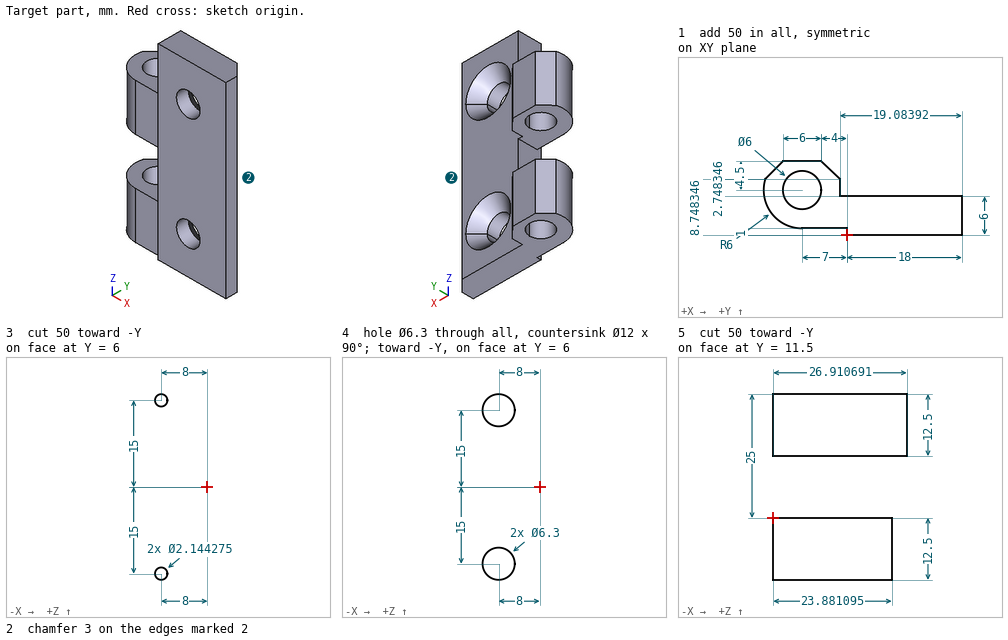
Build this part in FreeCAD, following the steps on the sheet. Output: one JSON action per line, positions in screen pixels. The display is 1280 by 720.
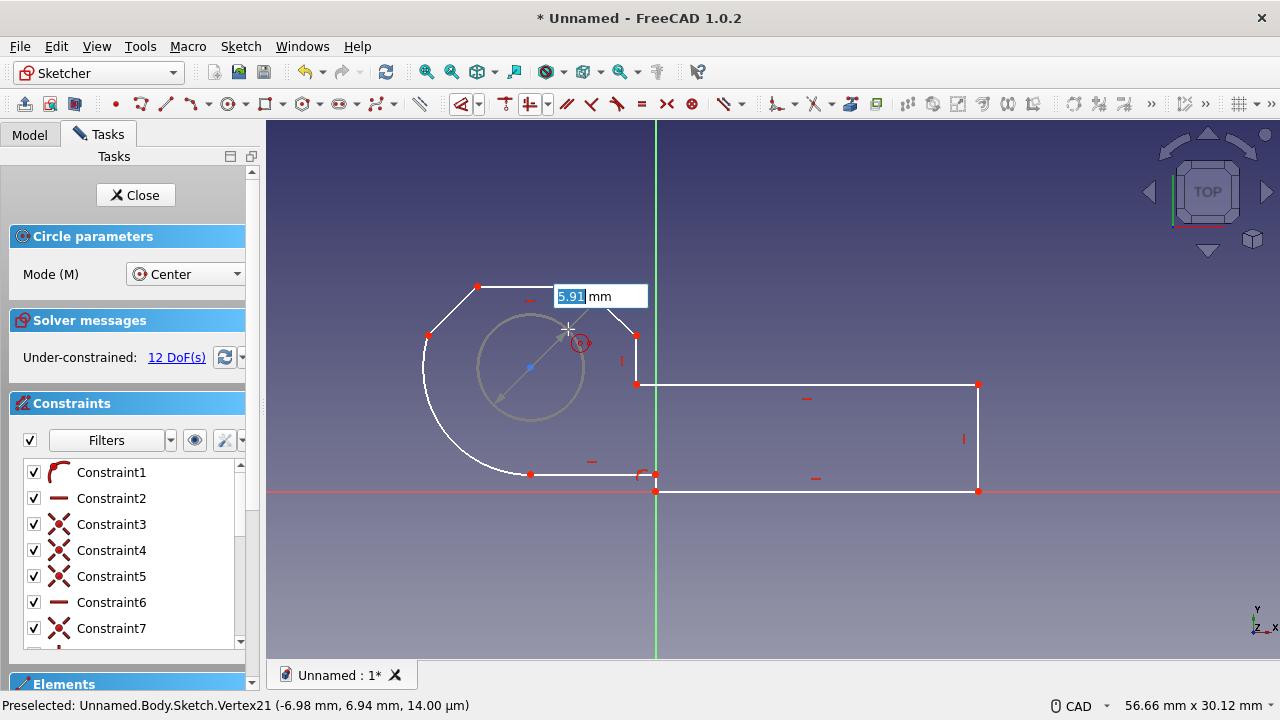
{"action": "type", "text": "6"}
{"action": "key", "text": "Return"}
{"action": "key", "text": "Escape"}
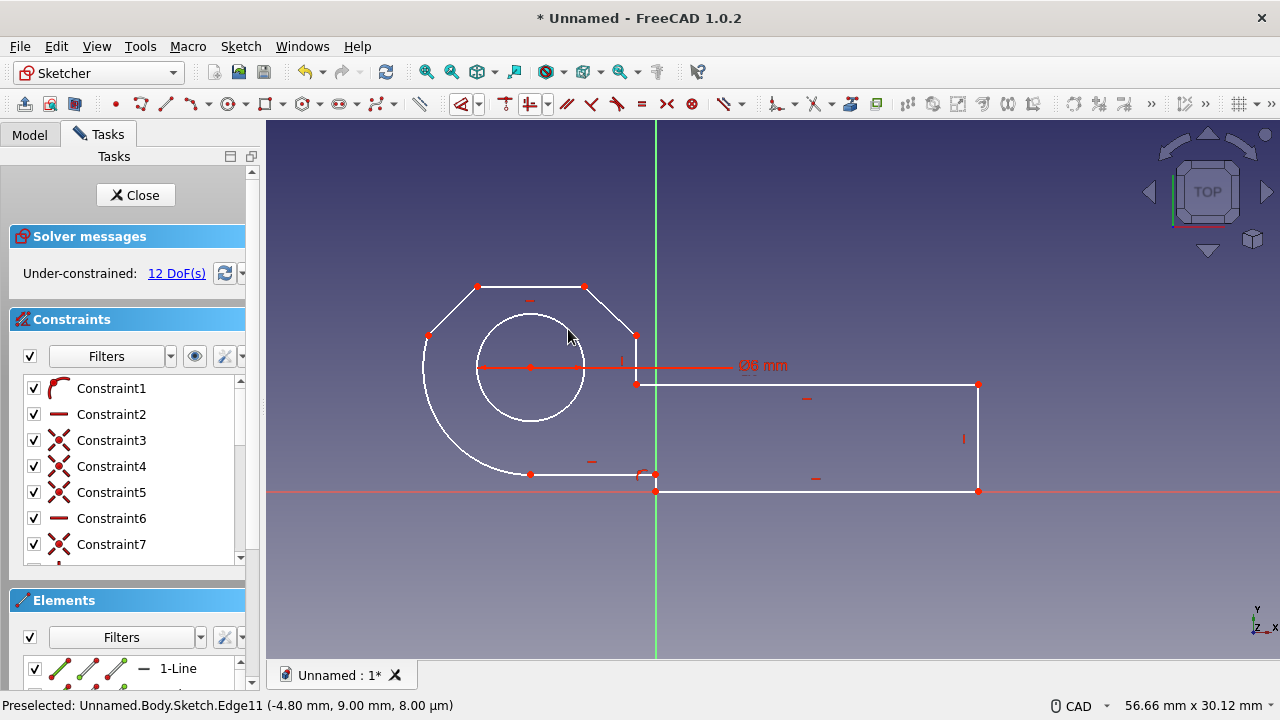
{"action": "left_click", "coordinate": [568, 475]}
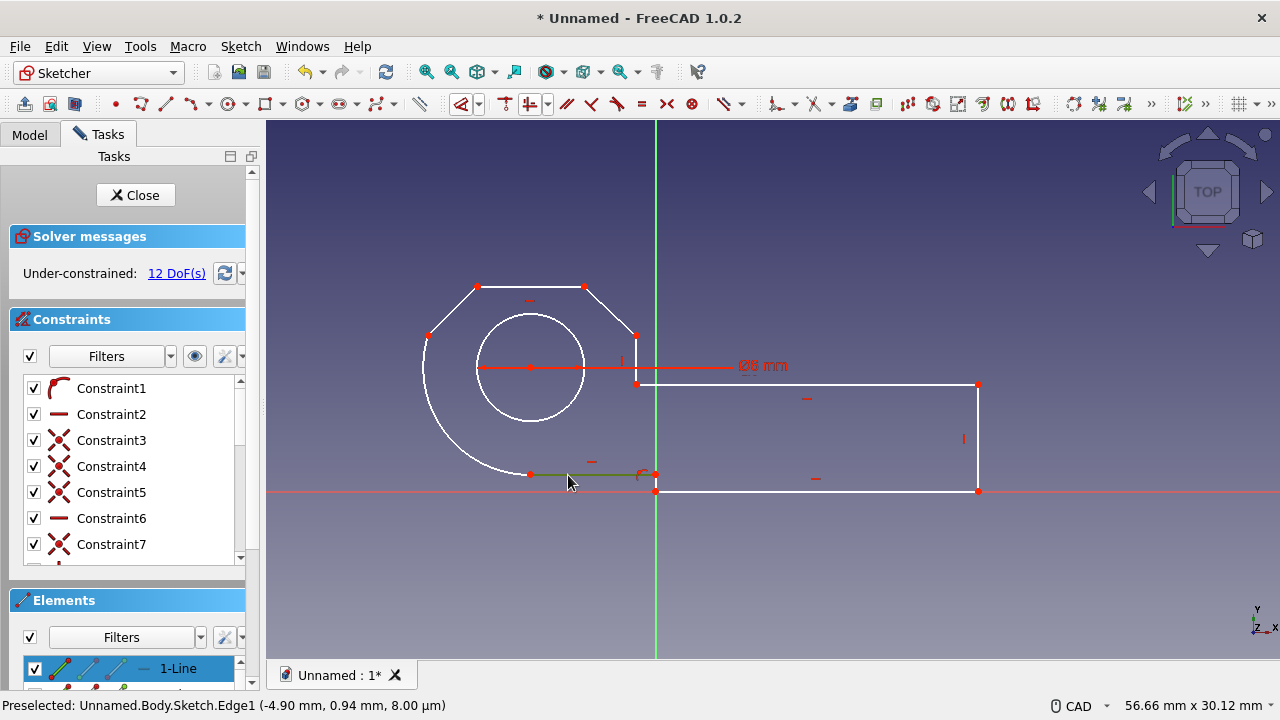
{"action": "left_click", "coordinate": [427, 395]}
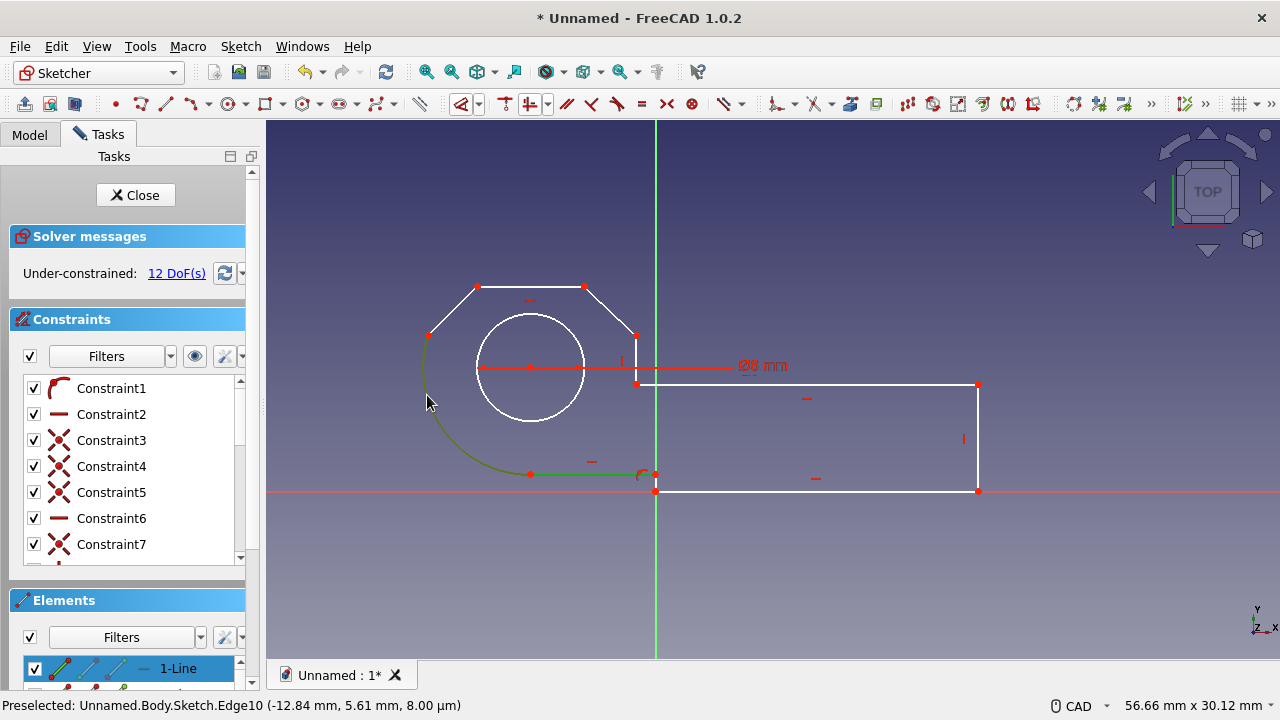
{"action": "left_click", "coordinate": [617, 104]}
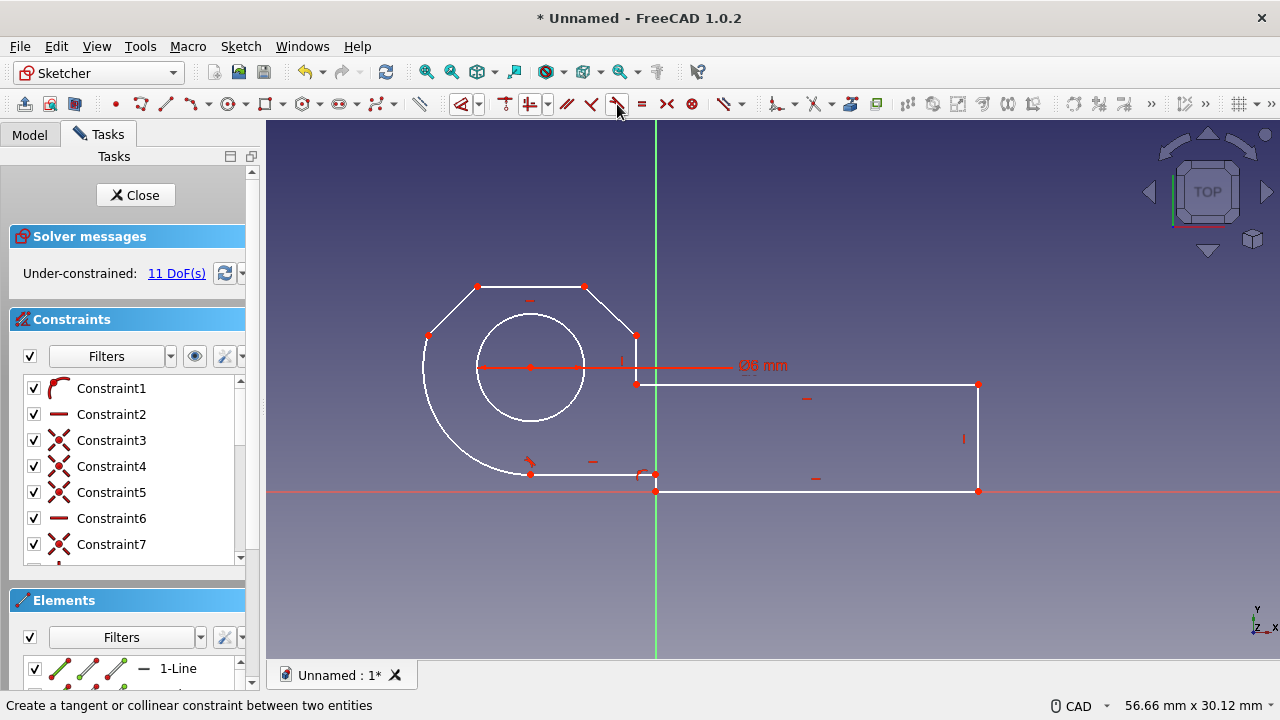
{"action": "left_click", "coordinate": [460, 104]}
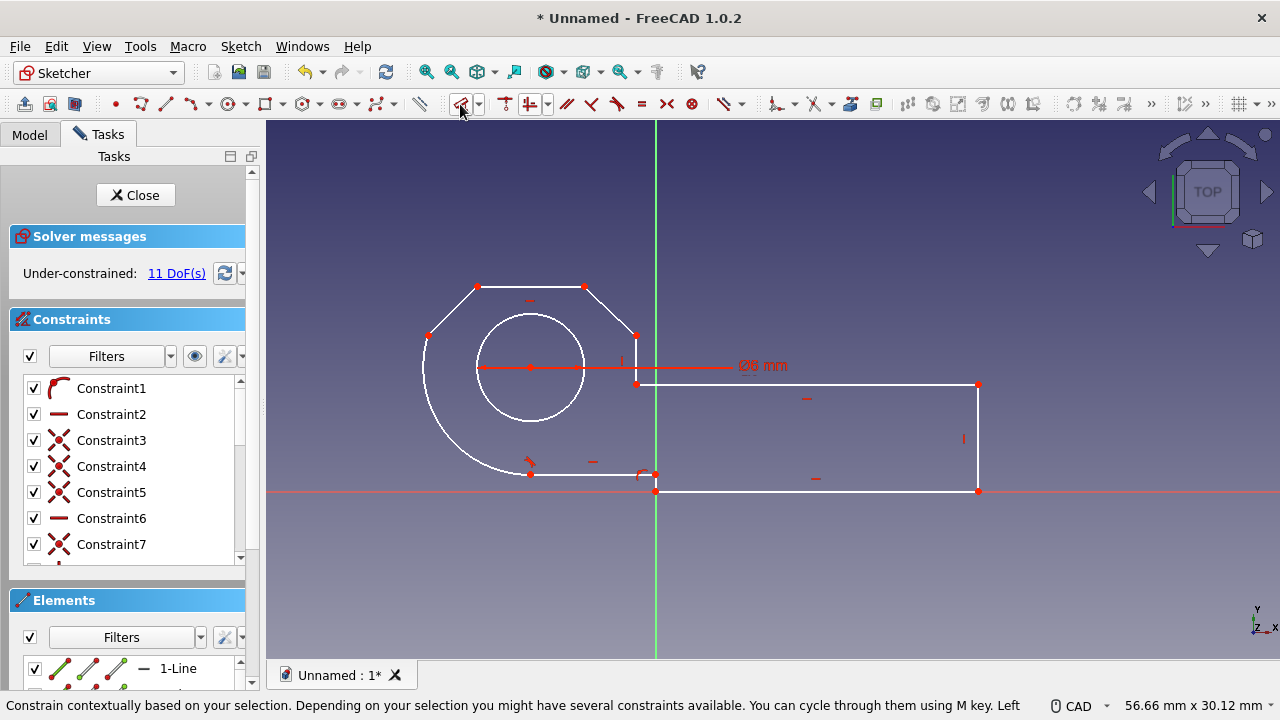
{"action": "left_click", "coordinate": [427, 395]}
{"action": "left_click", "coordinate": [396, 403]}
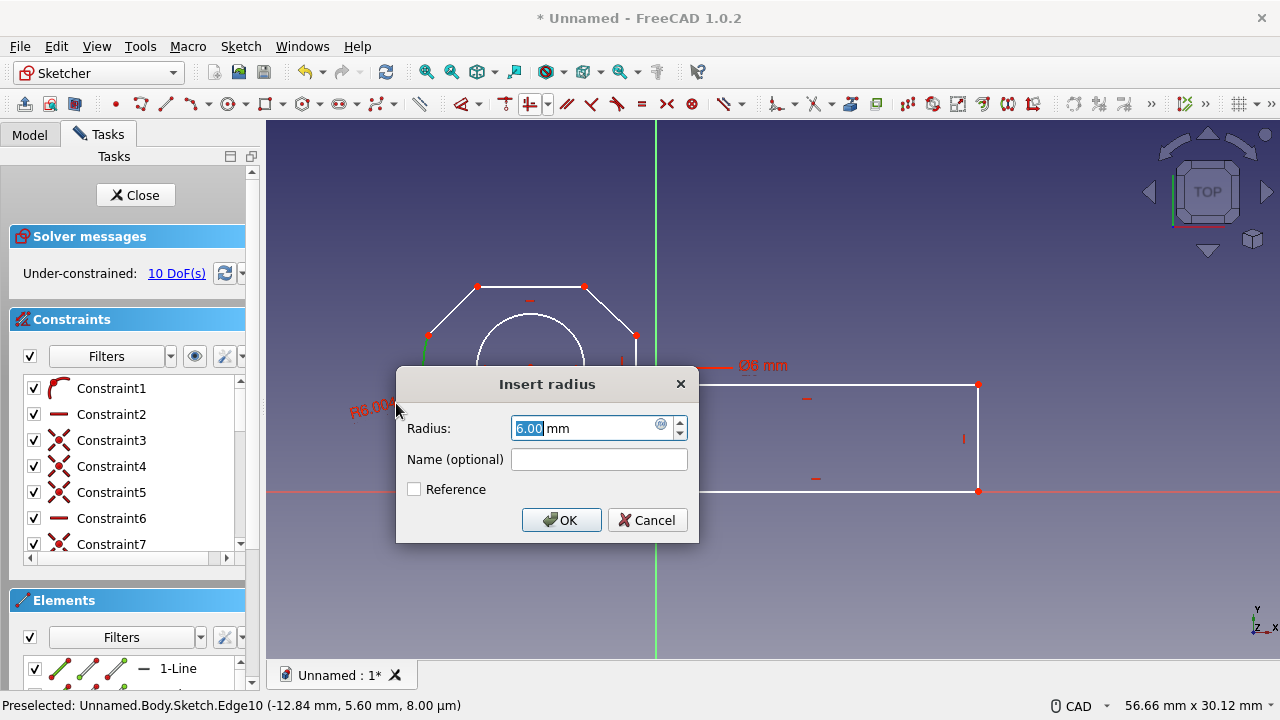
{"action": "type", "text": "6"}
{"action": "key", "text": "Return"}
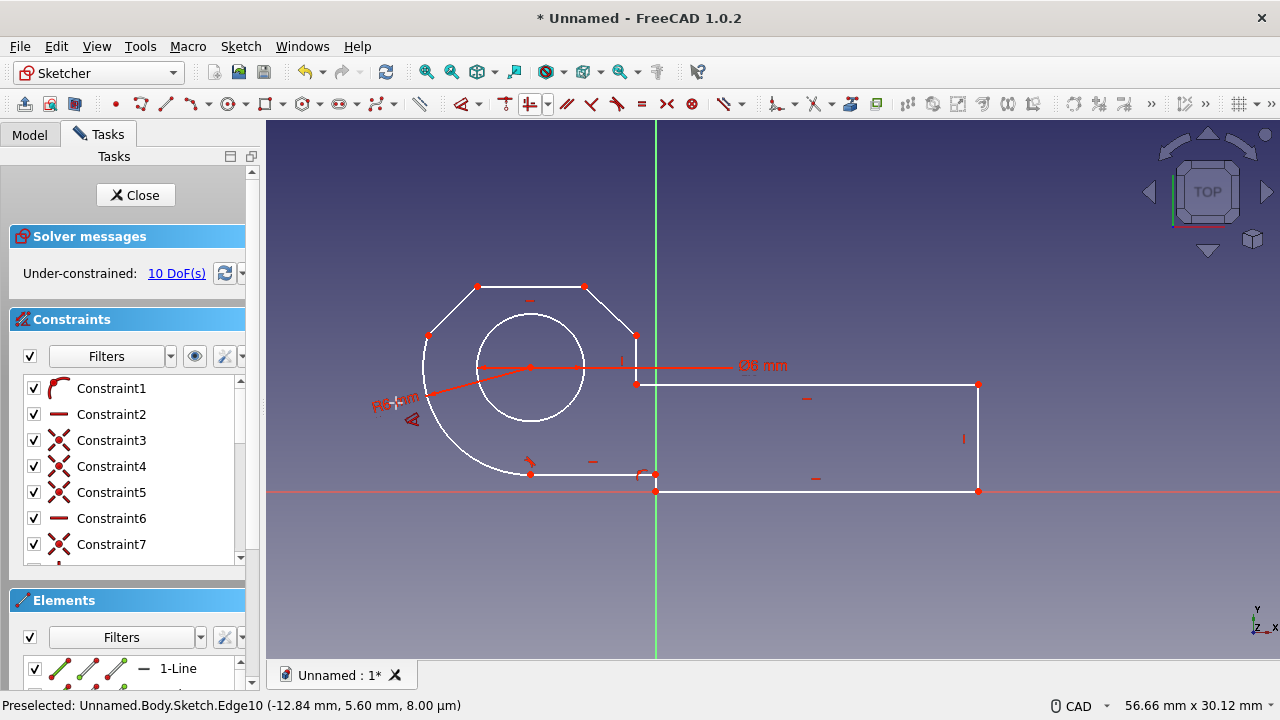
{"action": "left_click", "coordinate": [568, 475]}
{"action": "left_click", "coordinate": [593, 509]}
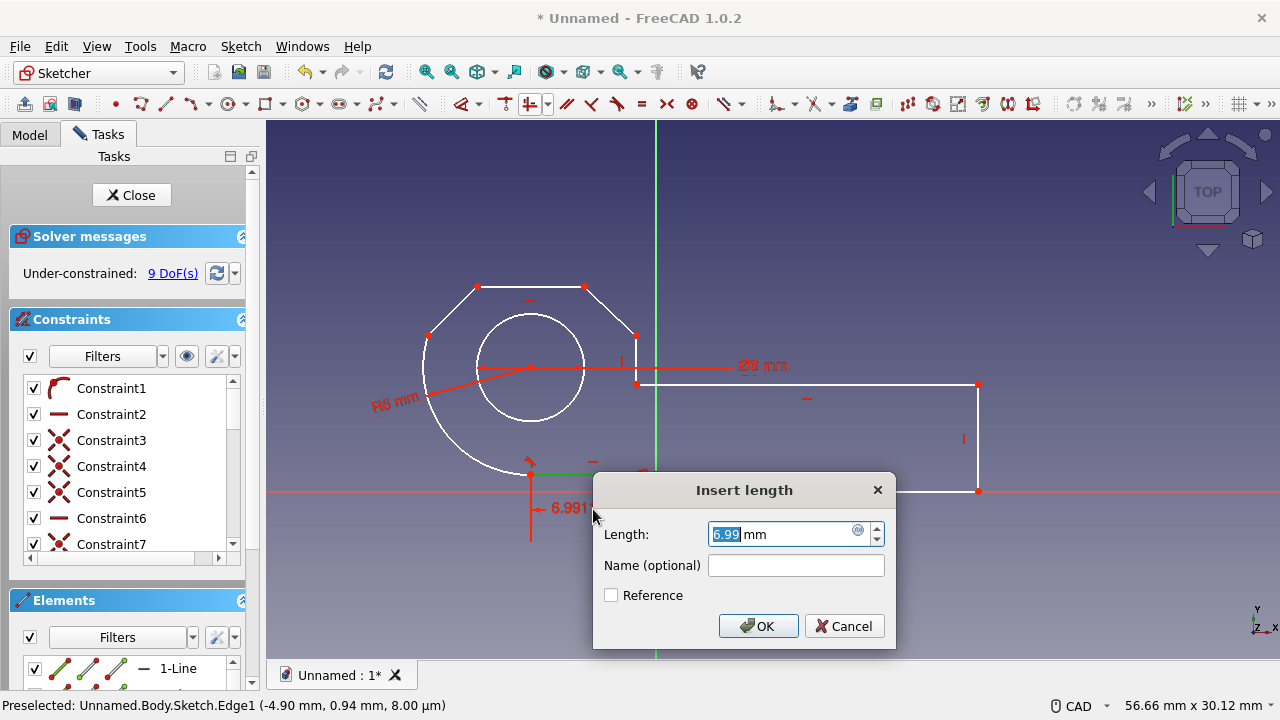
{"action": "type", "text": "7"}
{"action": "key", "text": "Return"}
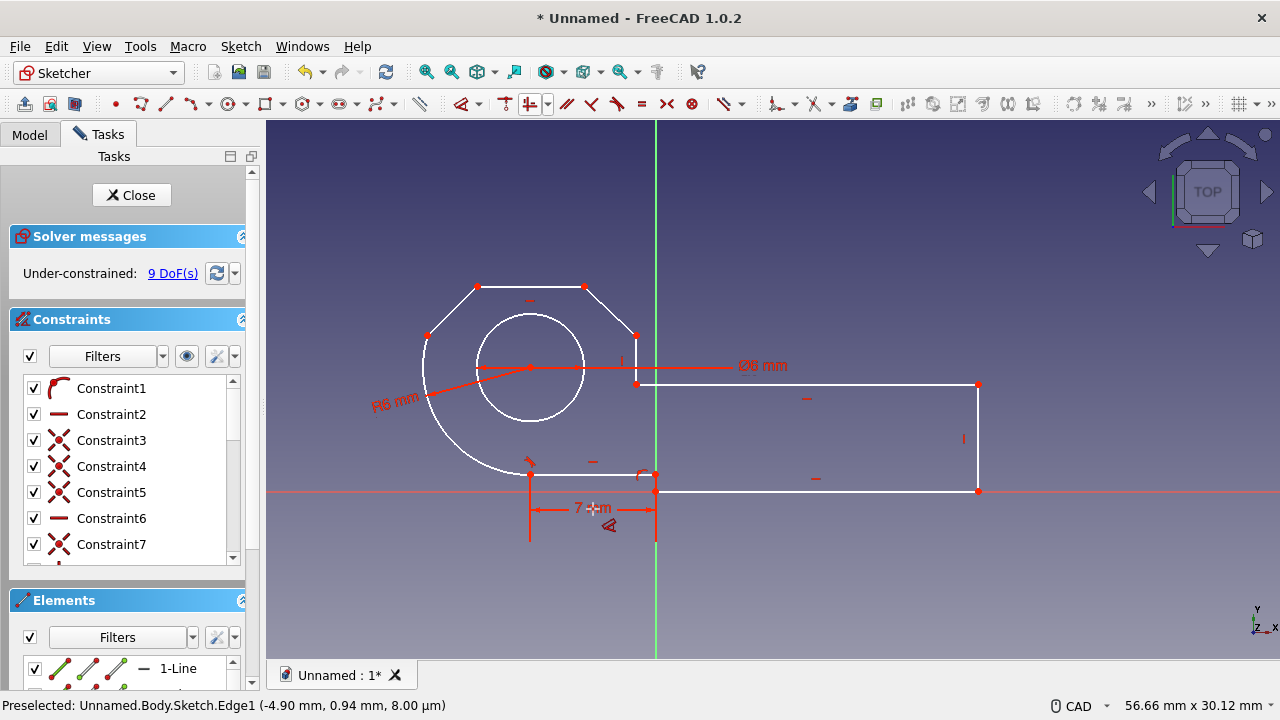
{"action": "scroll", "coordinate": [656, 483], "scroll_direction": "up", "scroll_amount": 4}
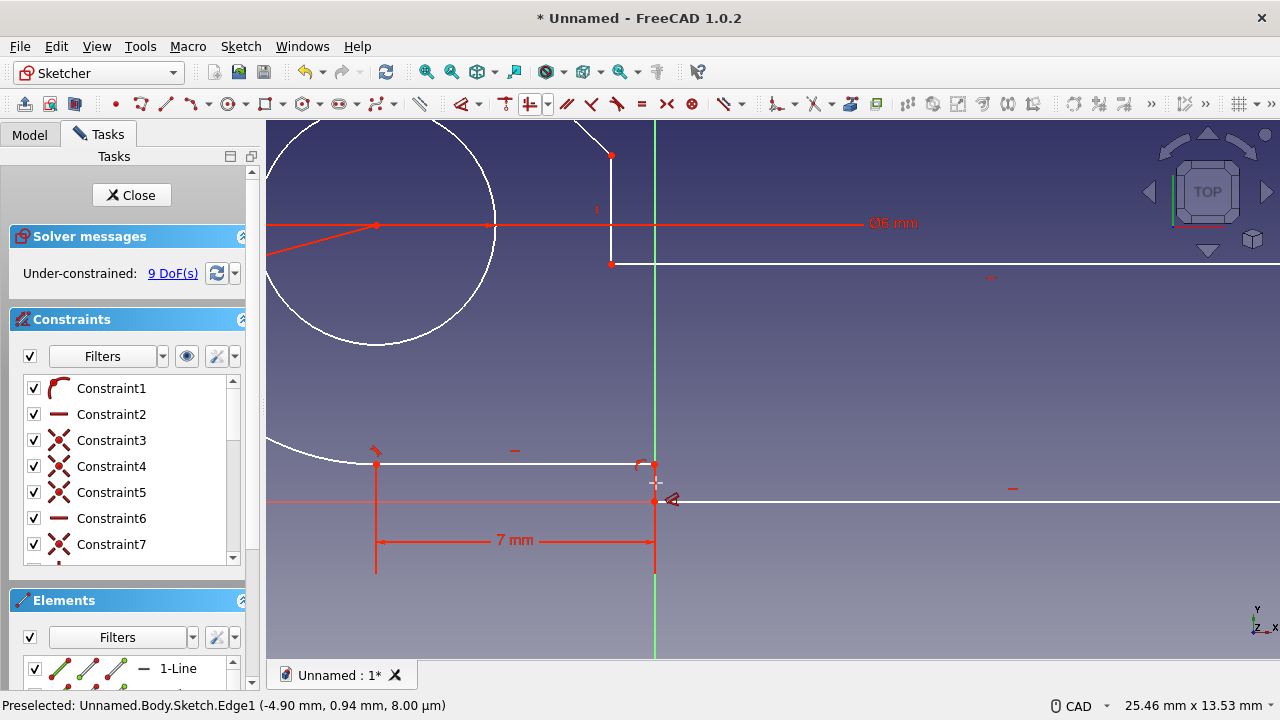
{"action": "left_click", "coordinate": [655, 483]}
{"action": "left_click", "coordinate": [621, 483]}